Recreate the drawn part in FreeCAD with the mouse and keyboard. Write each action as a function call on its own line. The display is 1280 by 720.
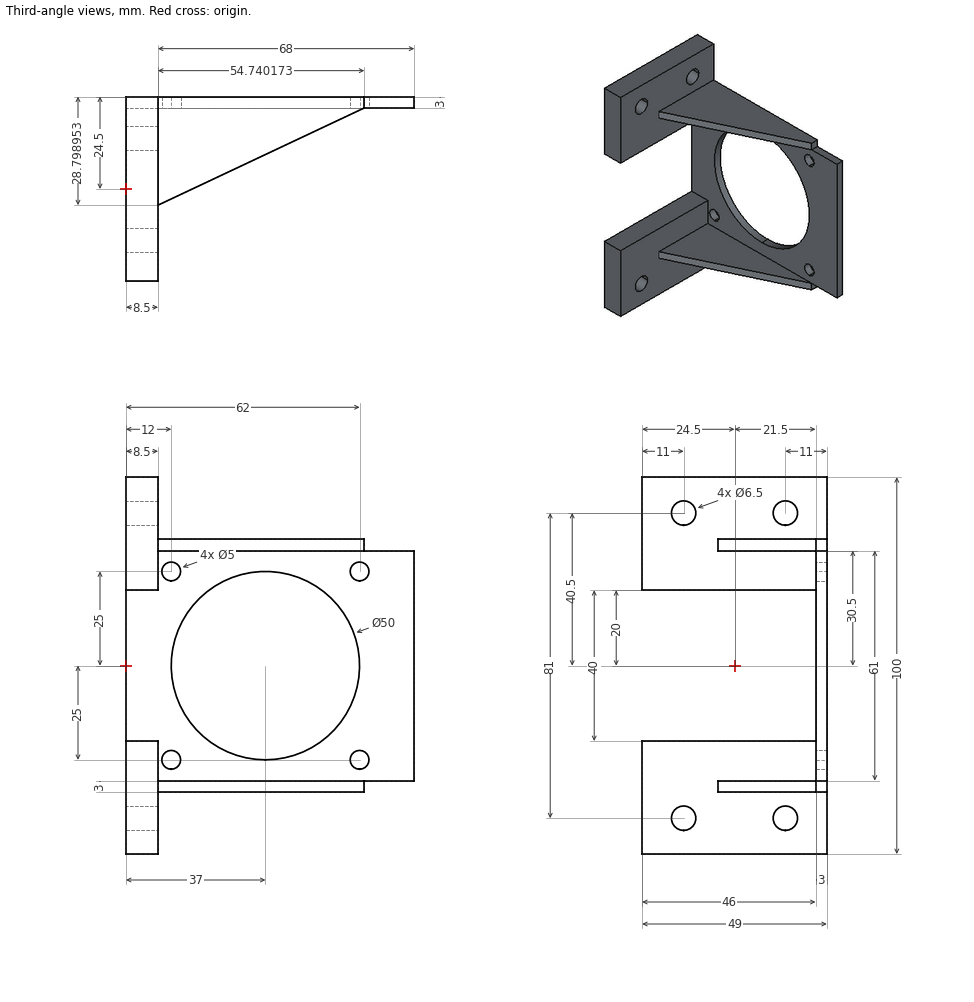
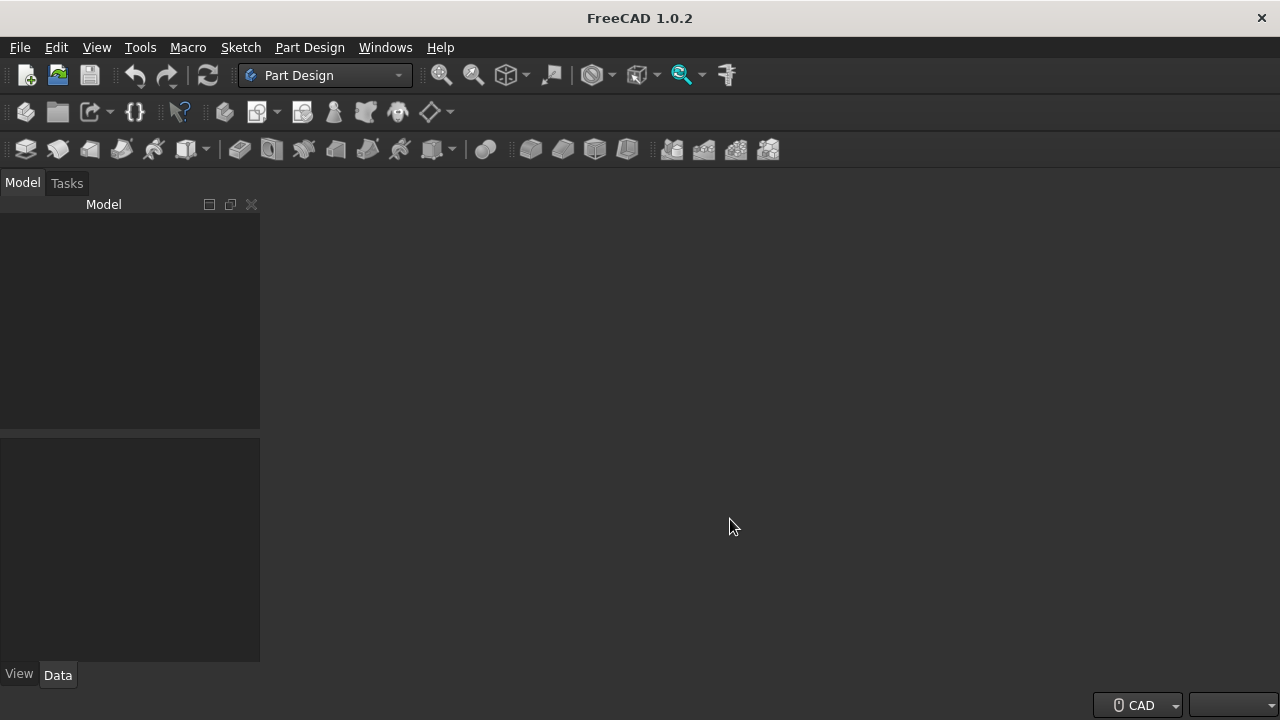
click(26, 76)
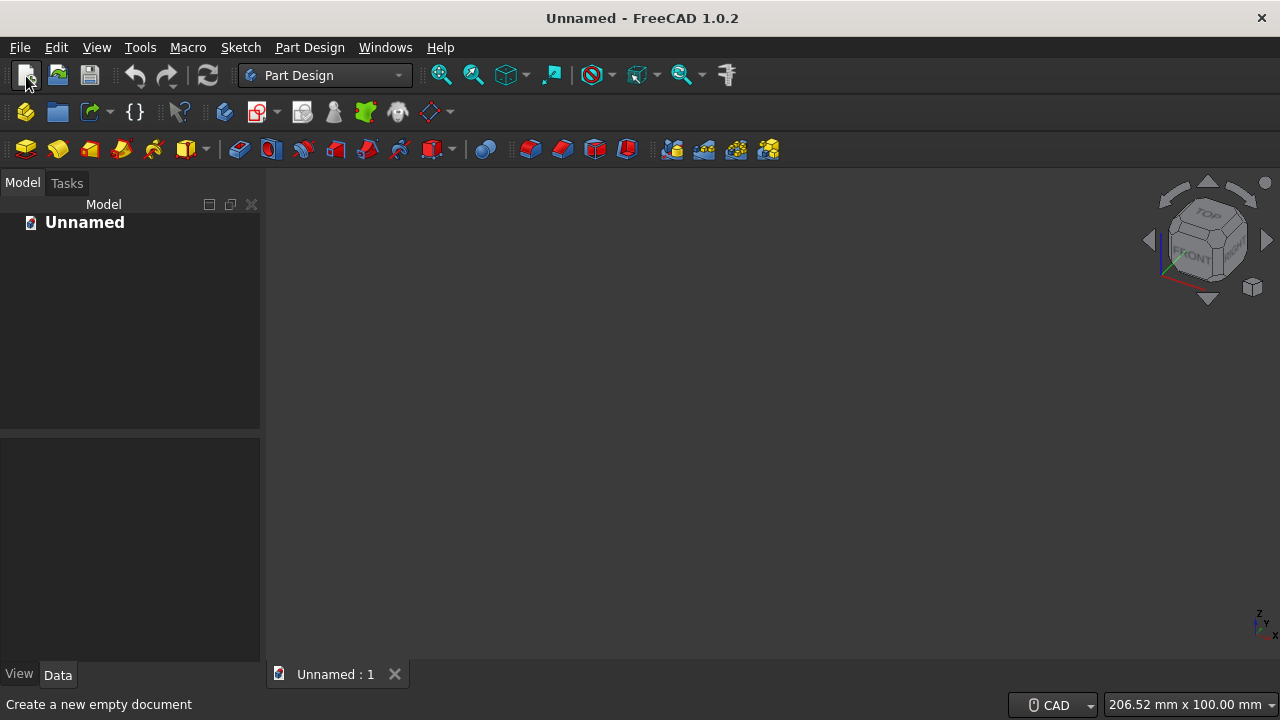
click(258, 112)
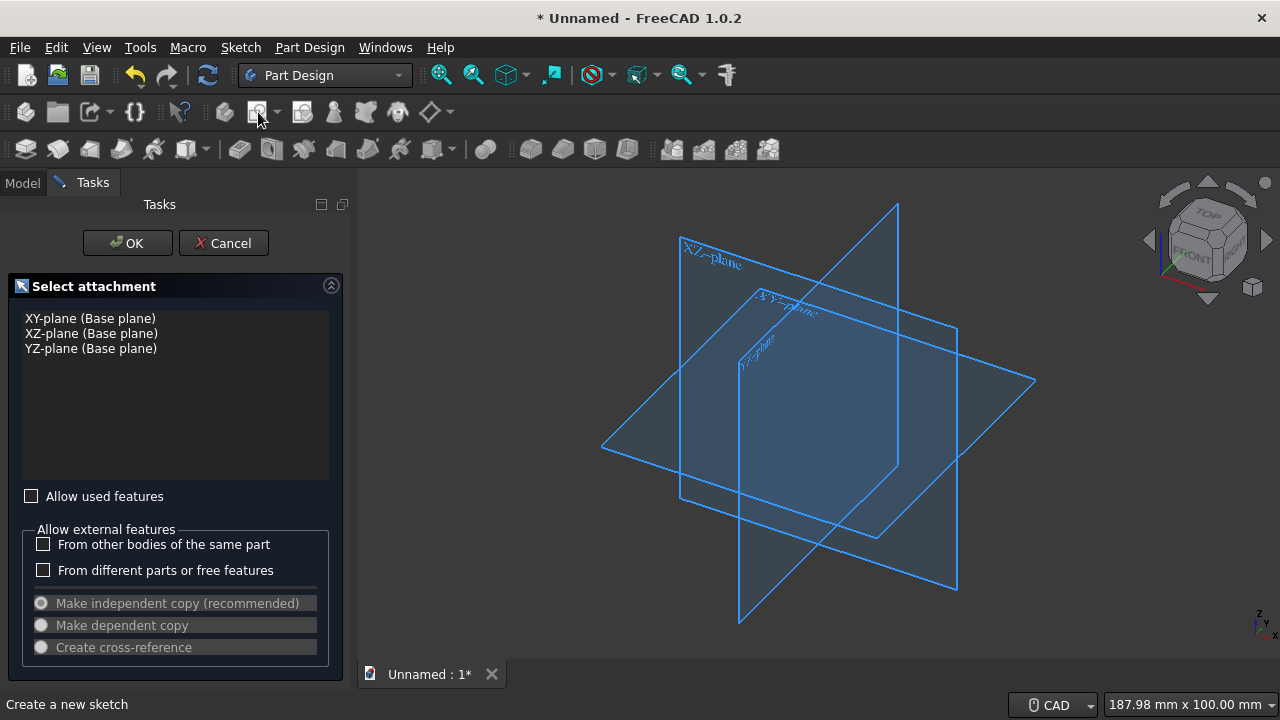
click(82, 348)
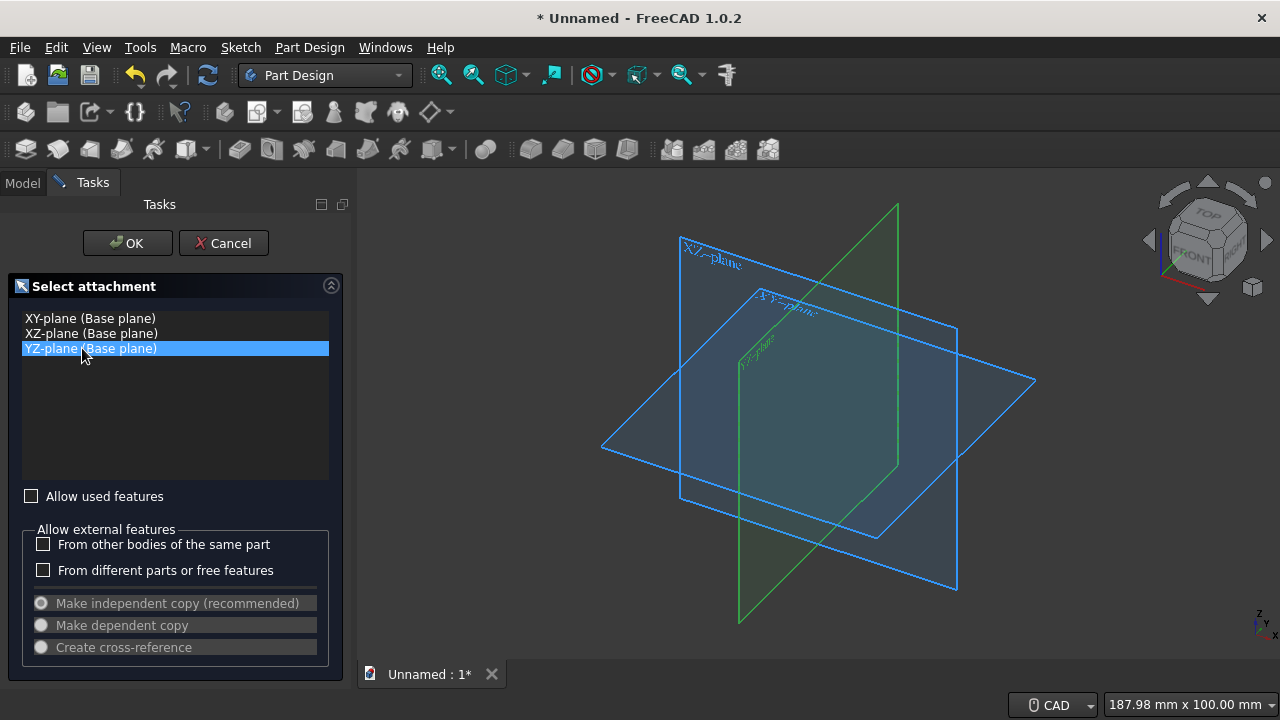
click(128, 243)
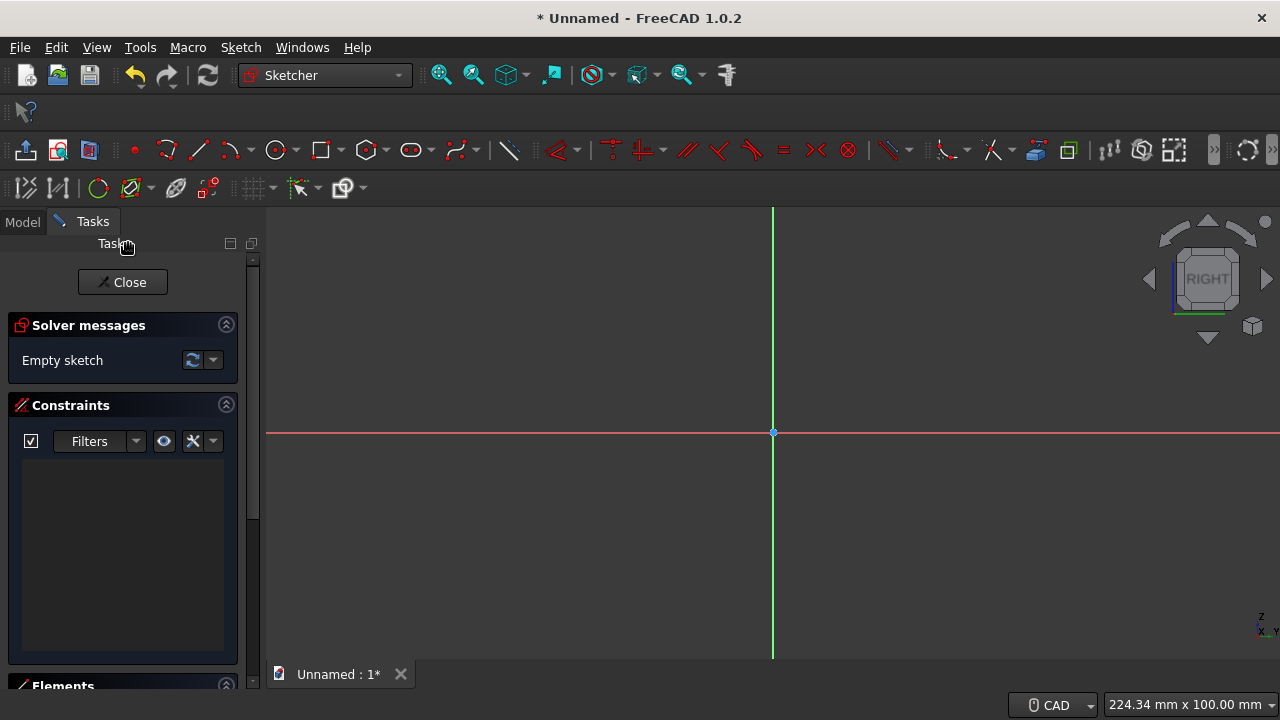
scroll(565, 433, down, 2)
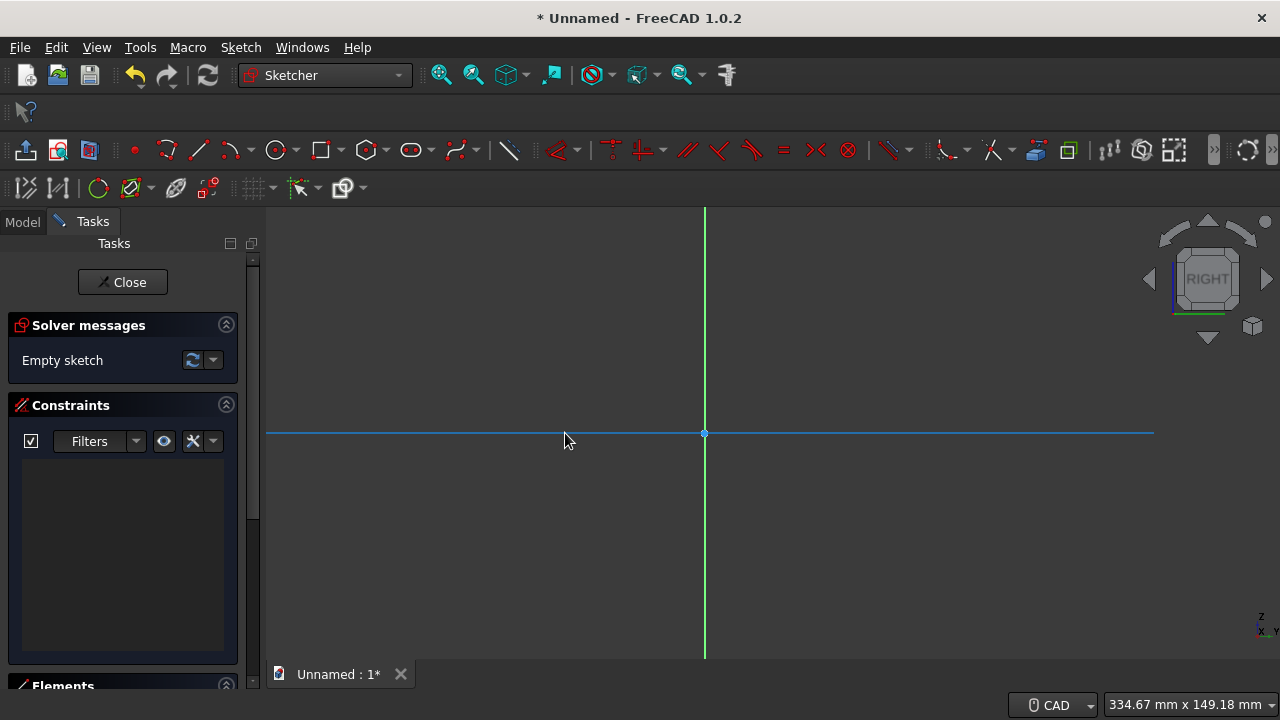
key(g)
key(v)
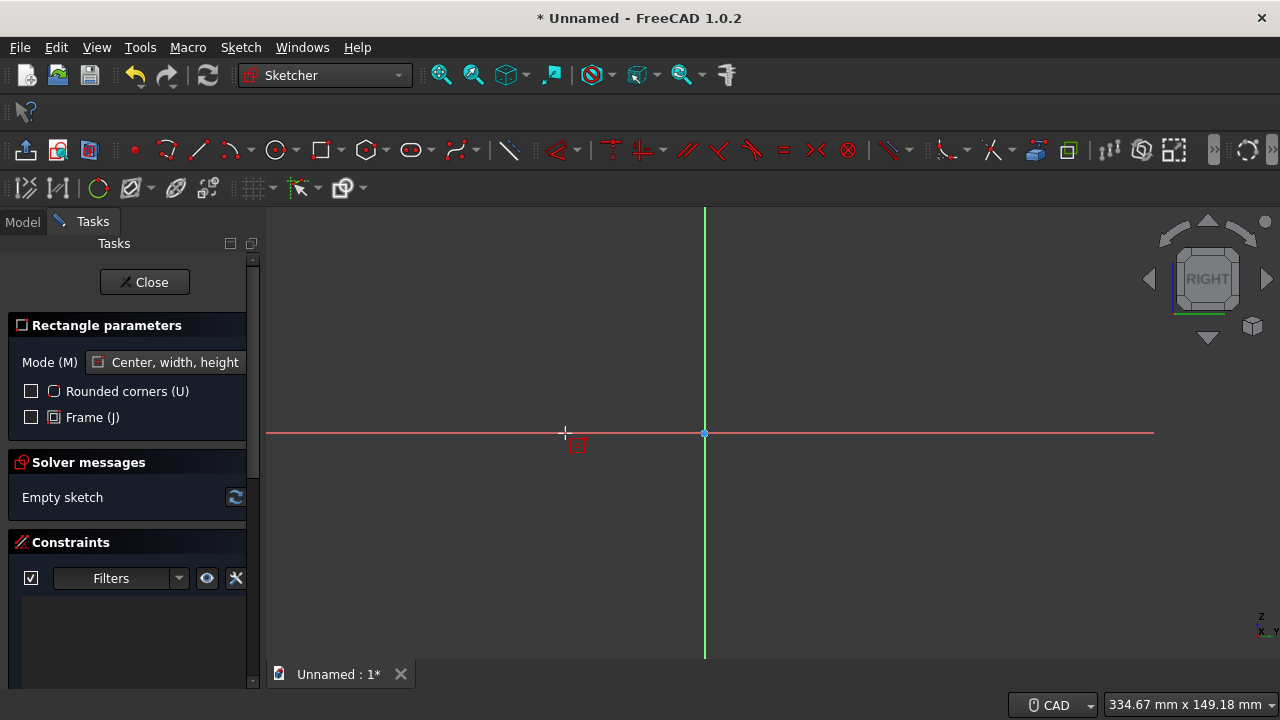
click(705, 433)
click(779, 282)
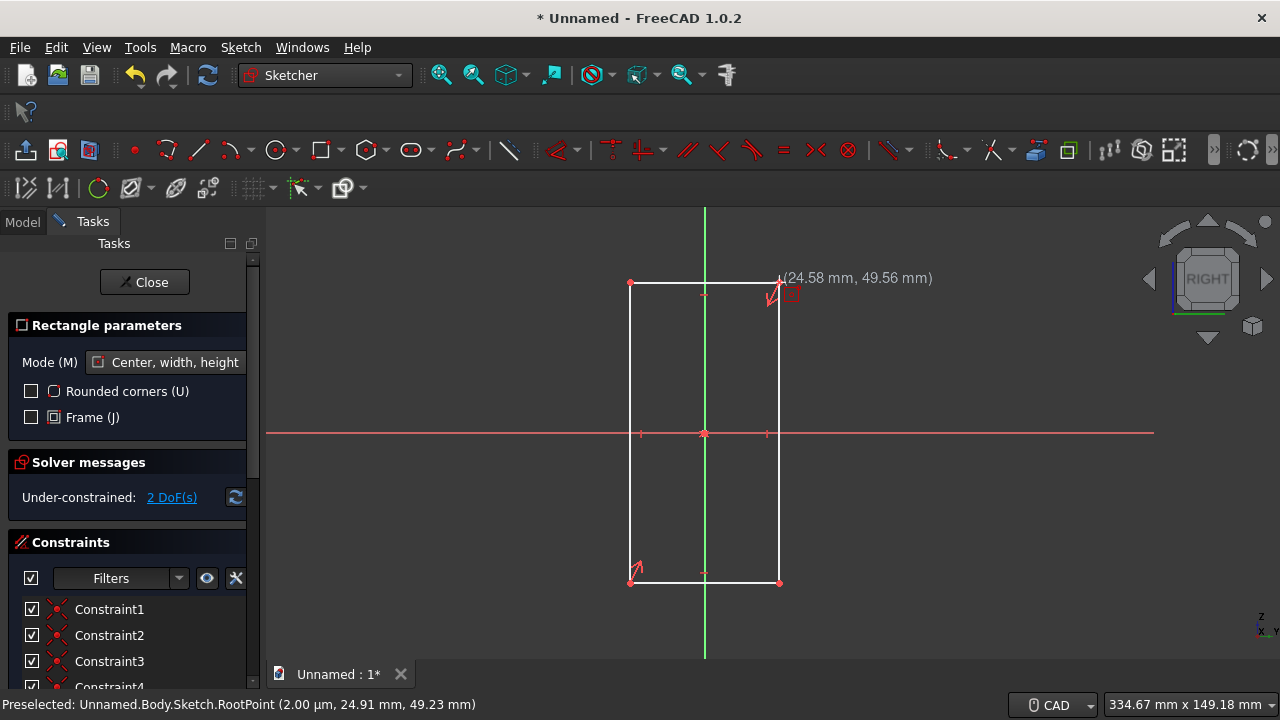
key(g)
key(c)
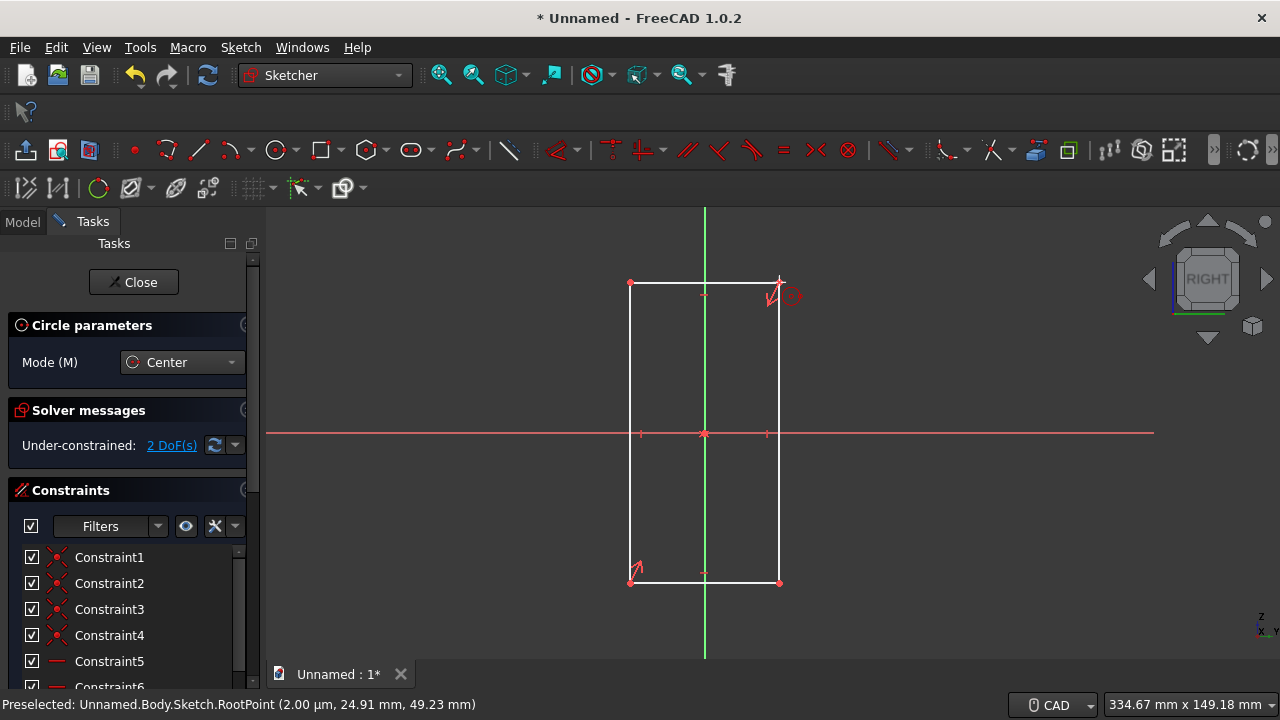
scroll(664, 310, up, 5)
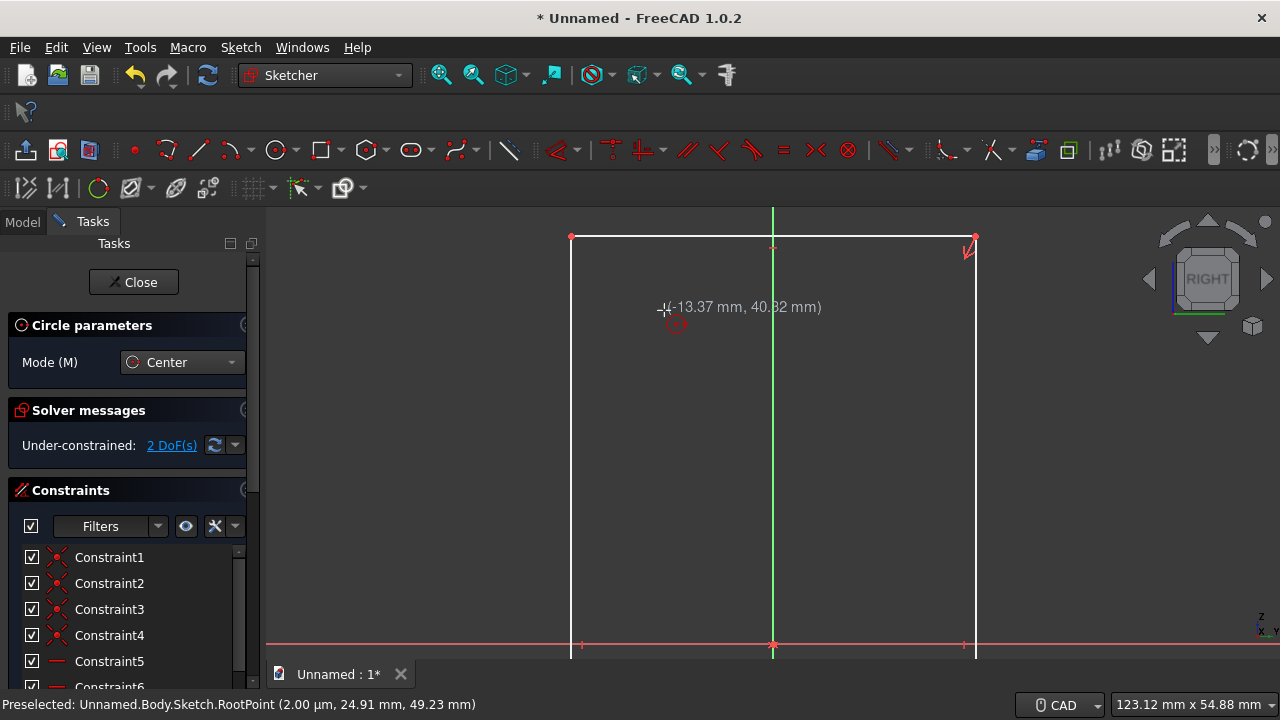
click(662, 311)
click(681, 292)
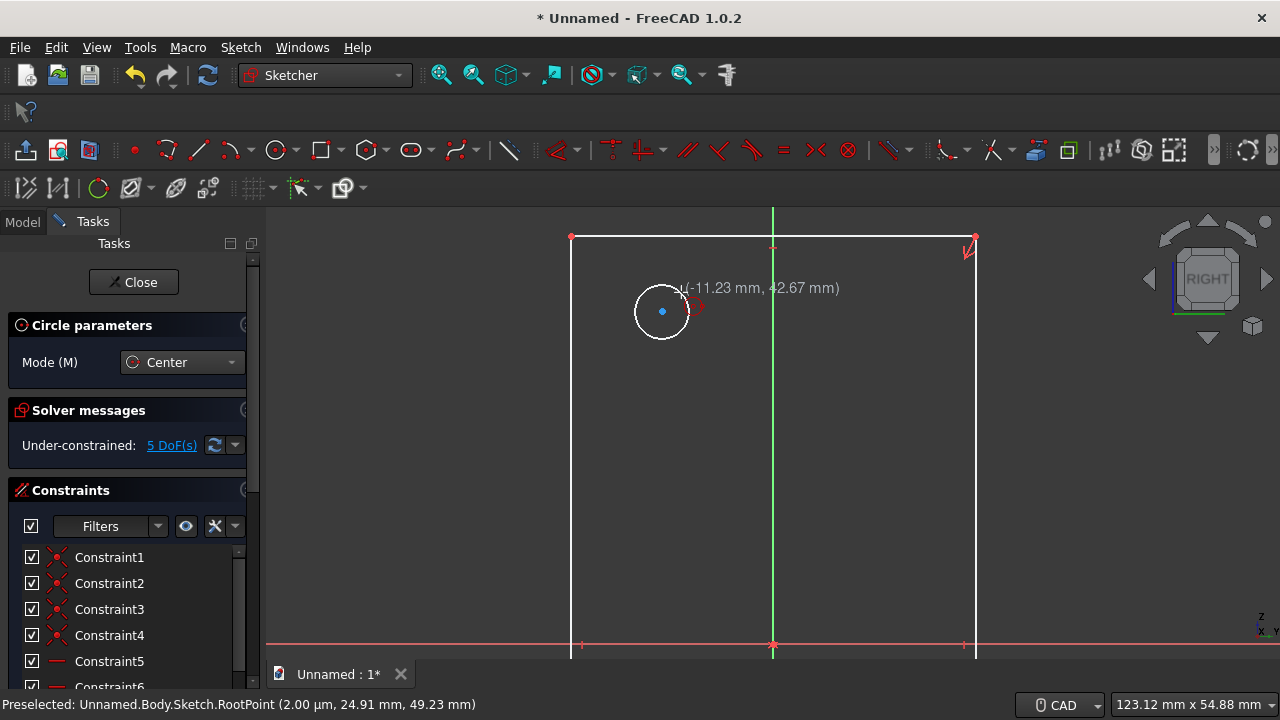
scroll(664, 310, down, 5)